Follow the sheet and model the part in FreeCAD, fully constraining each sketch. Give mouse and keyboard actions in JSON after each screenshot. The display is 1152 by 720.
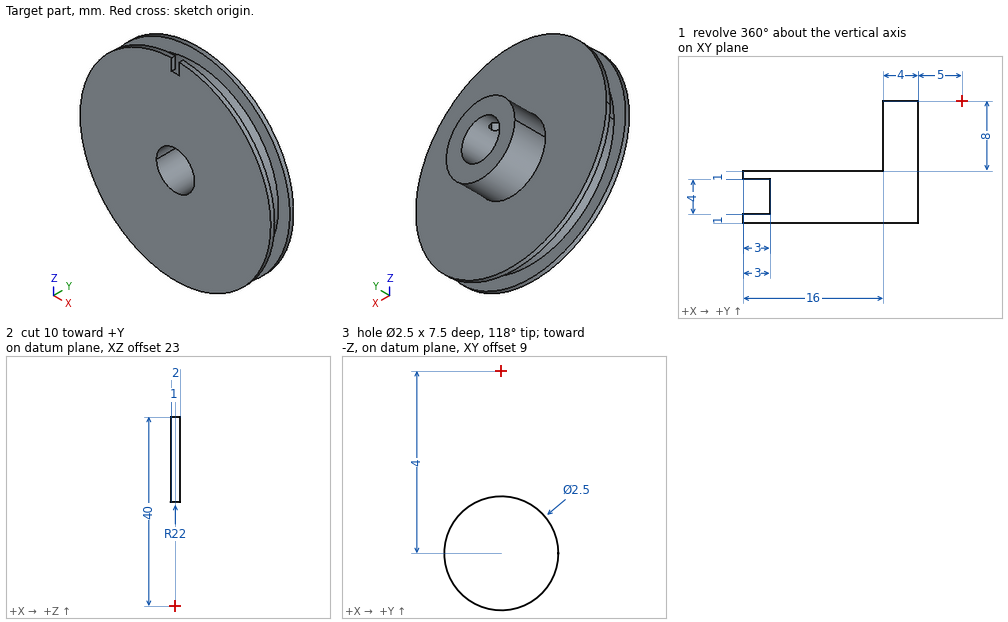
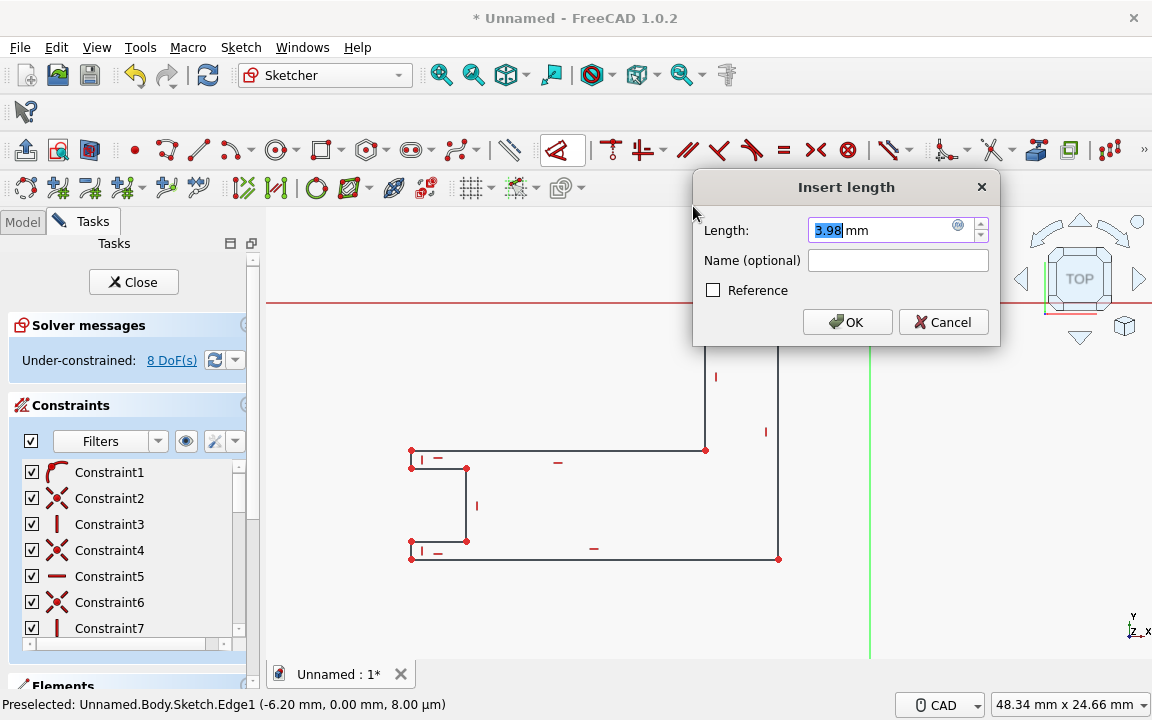
{"action": "type", "text": "4"}
{"action": "key", "text": "Return"}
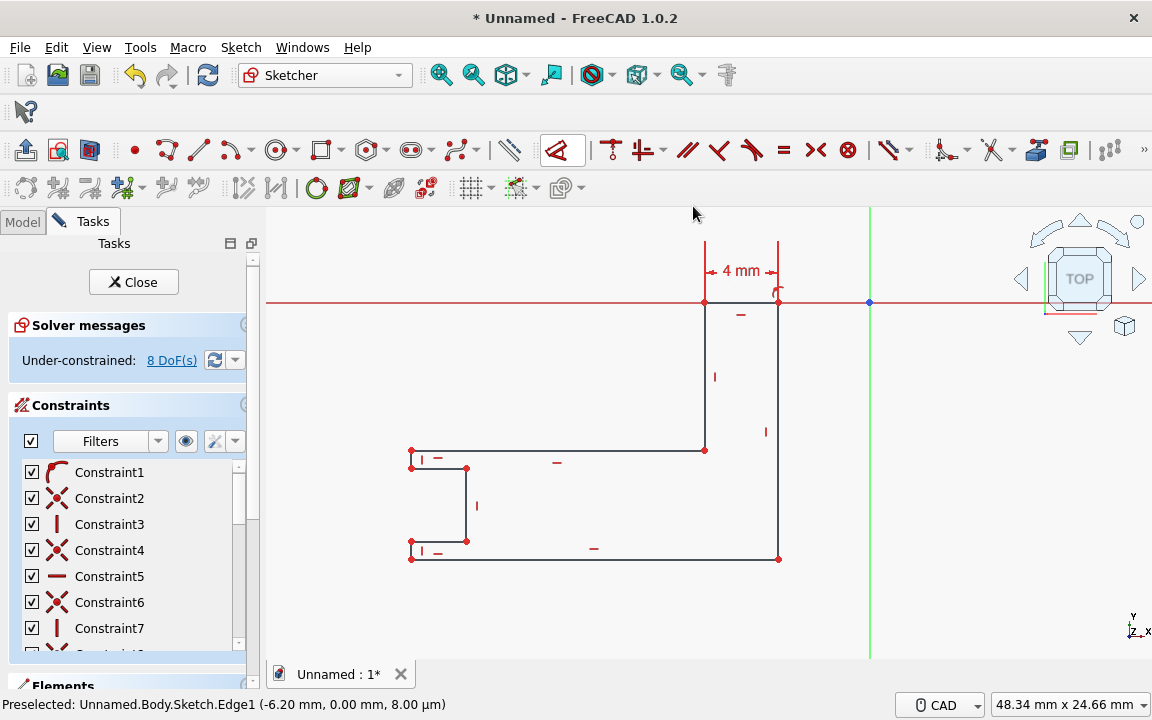
{"action": "left_click", "coordinate": [705, 347]}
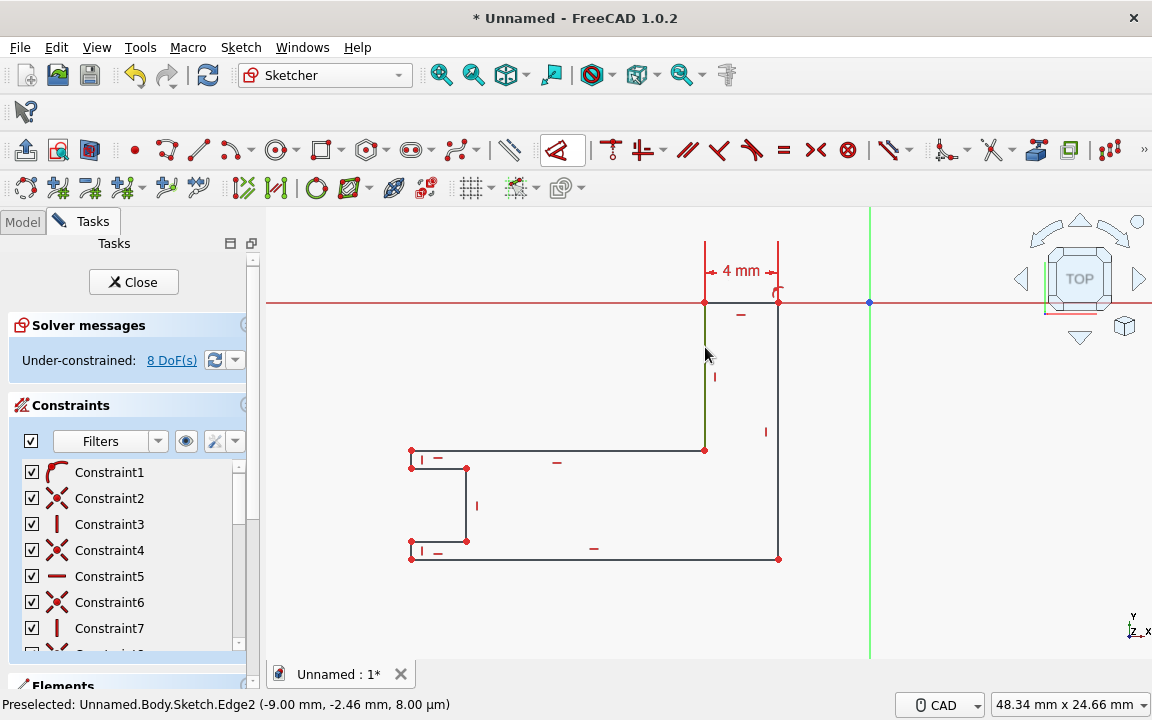
{"action": "key", "text": "i"}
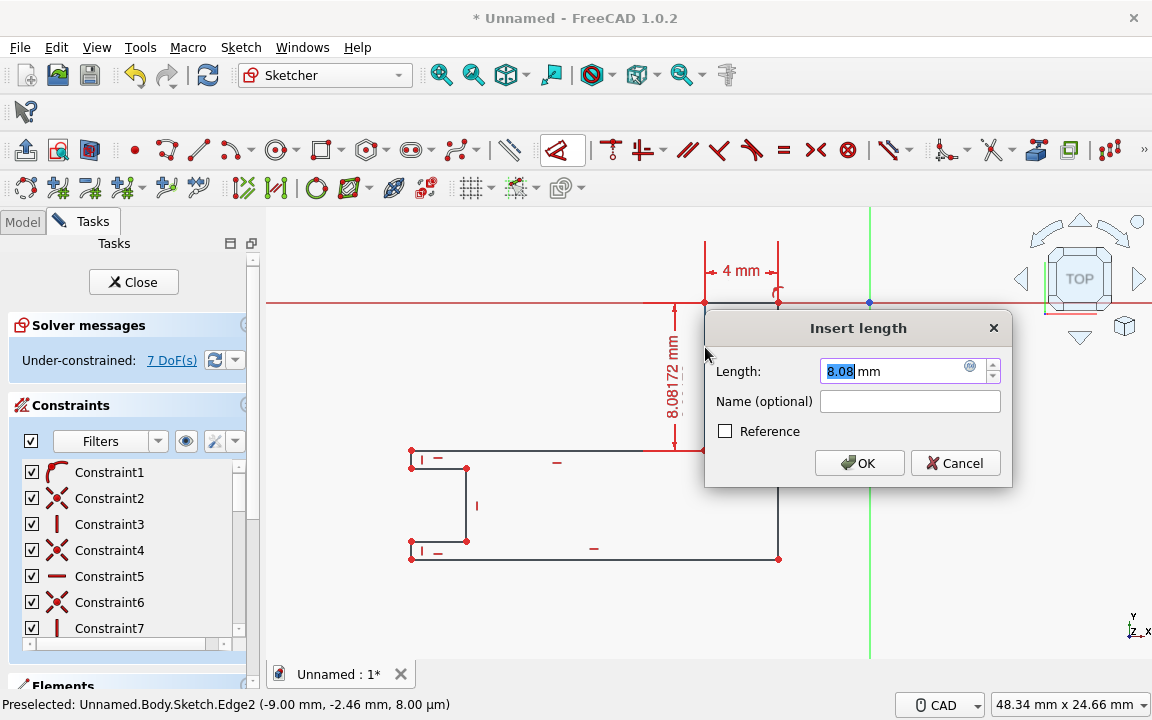
{"action": "type", "text": "8"}
{"action": "key", "text": "Return"}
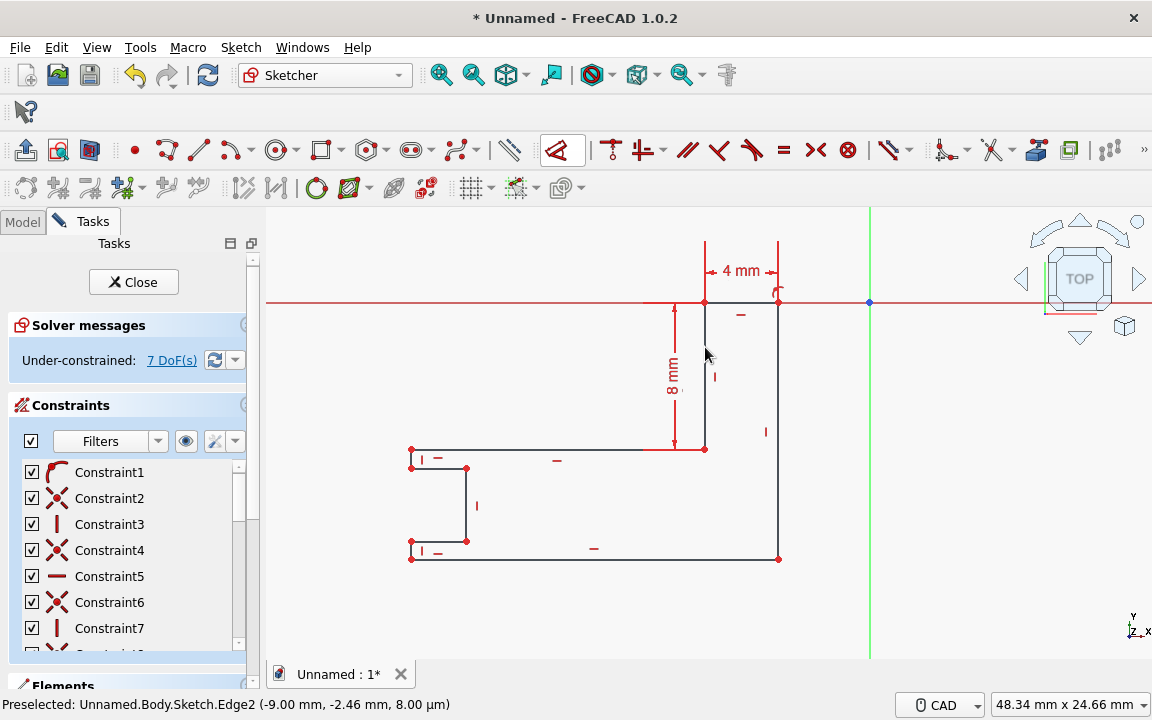
{"action": "scroll", "coordinate": [411, 459], "scroll_direction": "up", "scroll_amount": 4}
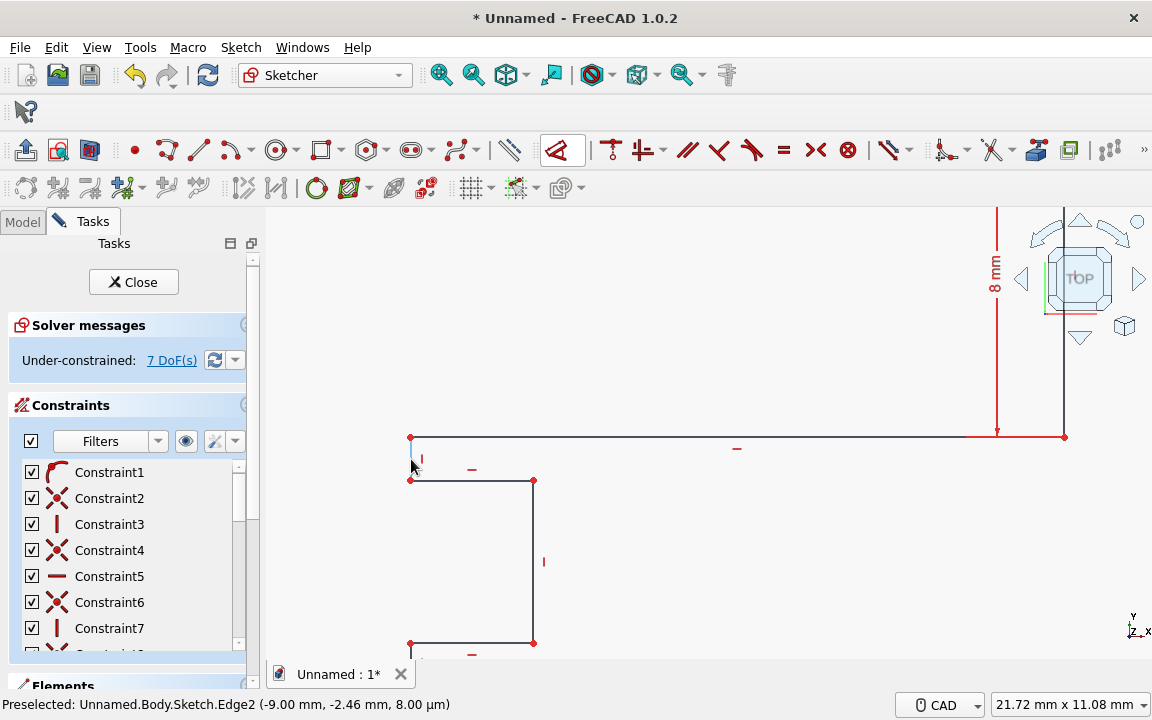
{"action": "left_click", "coordinate": [411, 459]}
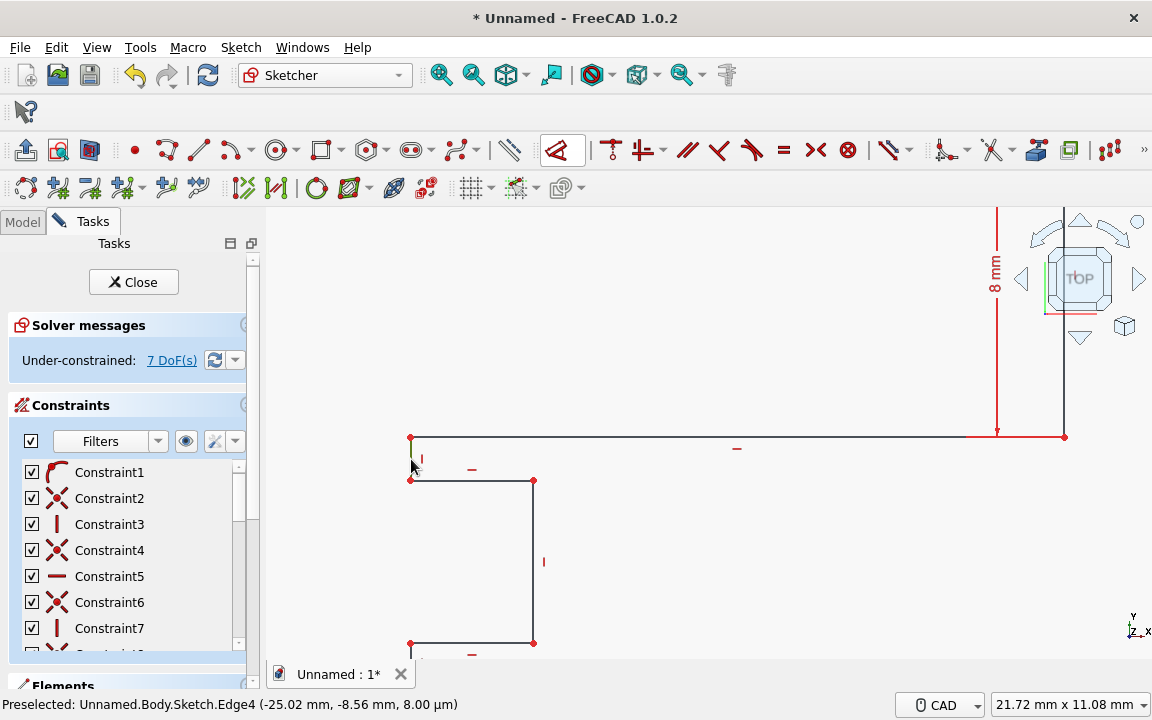
{"action": "key", "text": "i"}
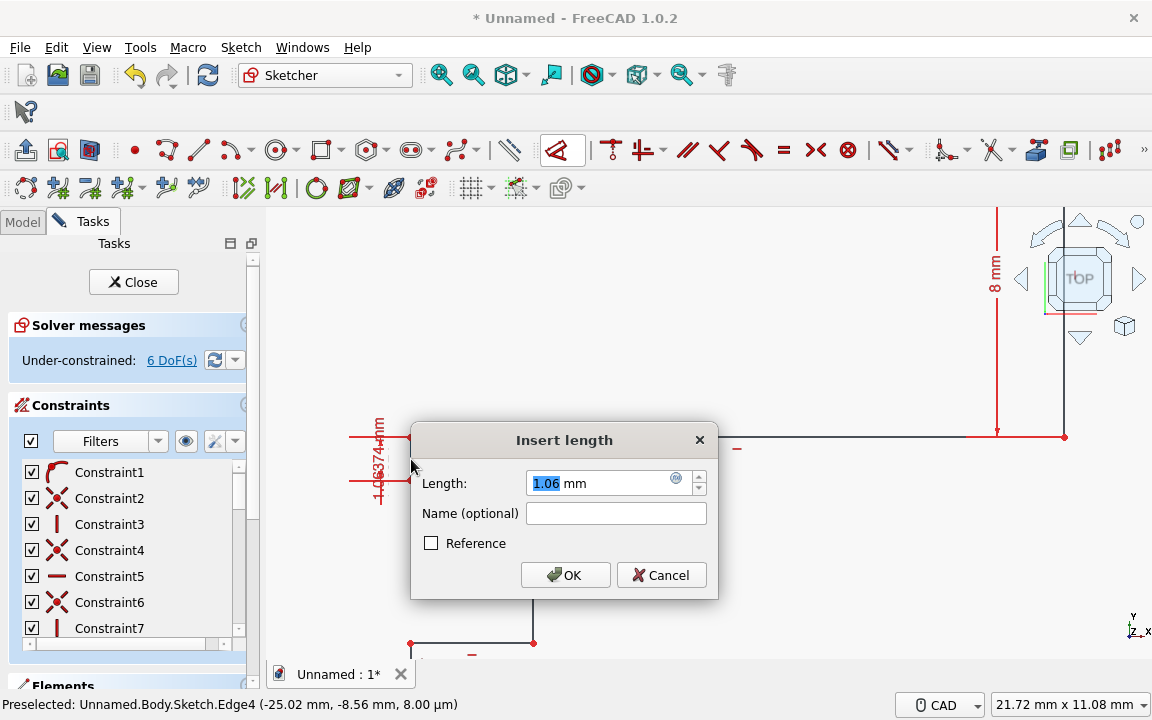
{"action": "type", "text": "1"}
{"action": "key", "text": "Return"}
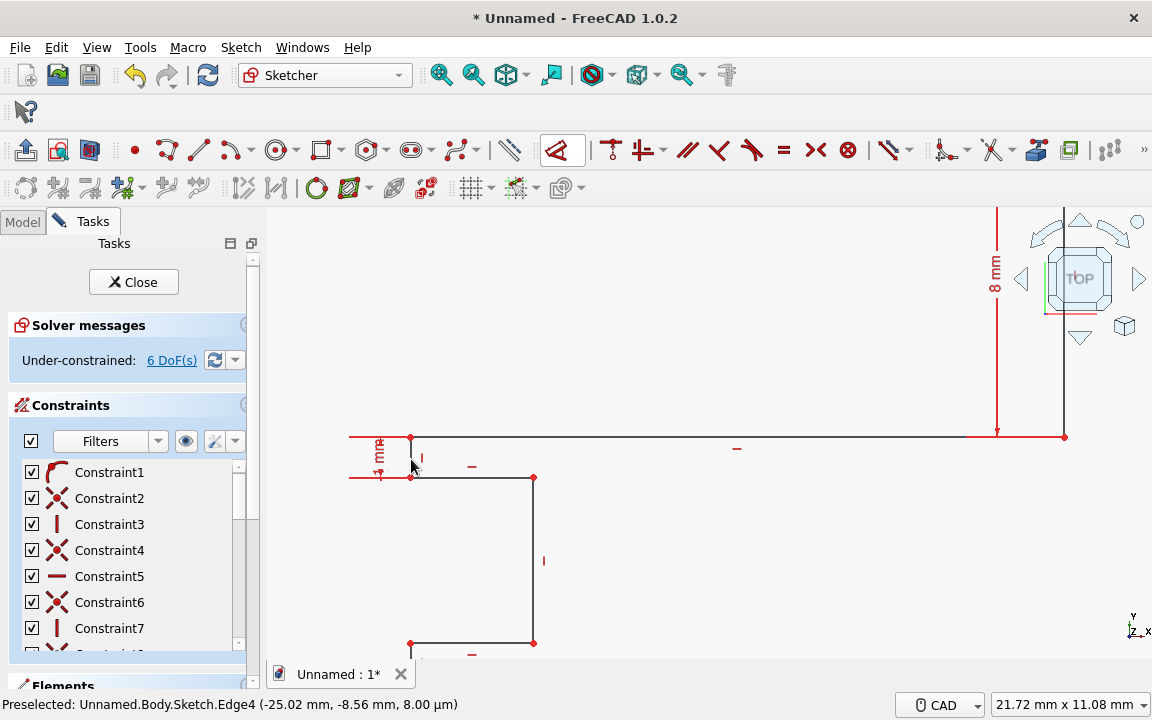
{"action": "left_click", "coordinate": [448, 478]}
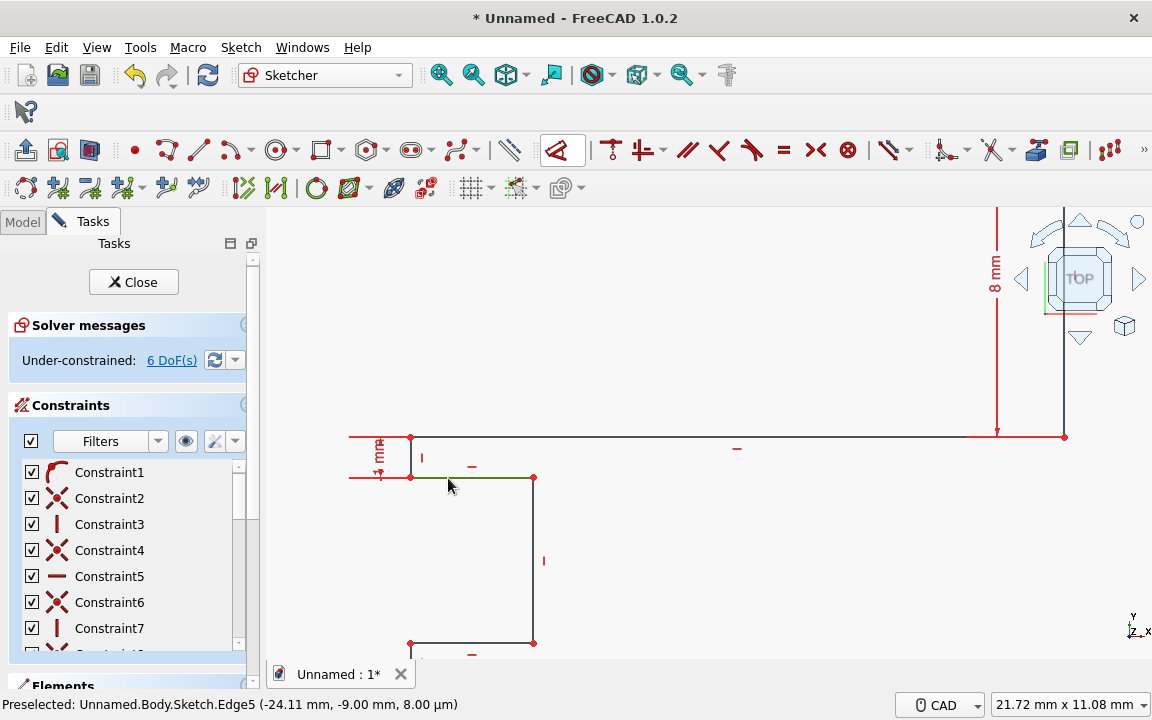
{"action": "key", "text": "l"}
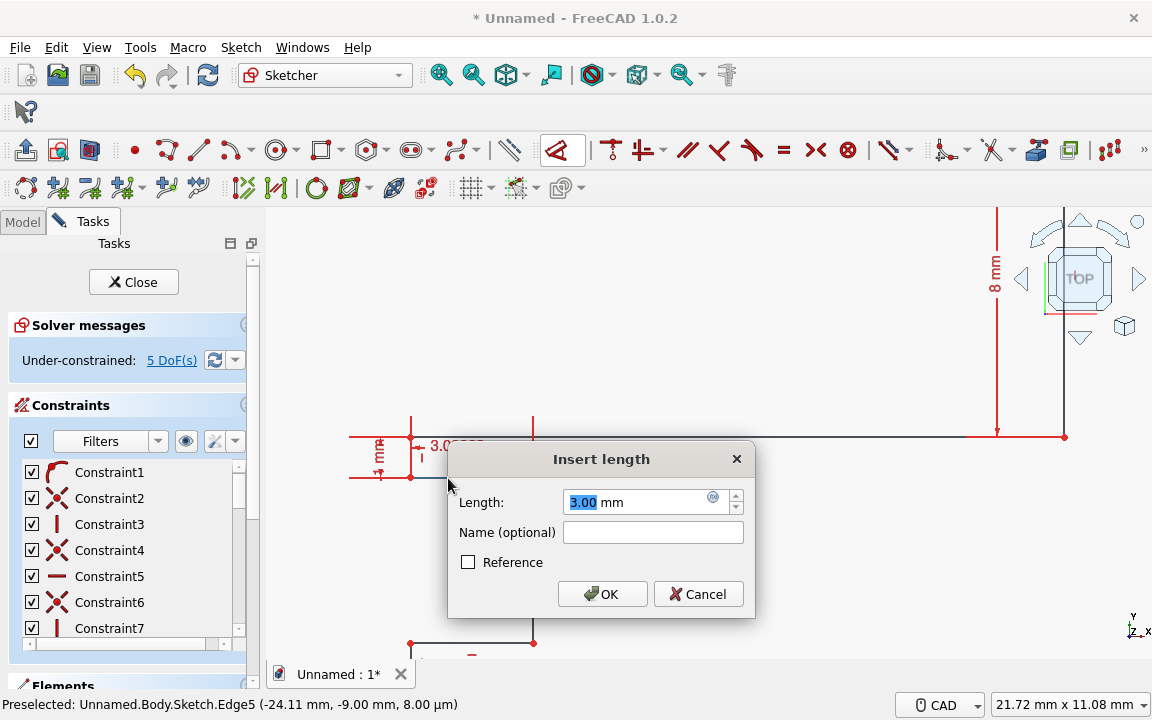
{"action": "type", "text": "3"}
{"action": "key", "text": "Return"}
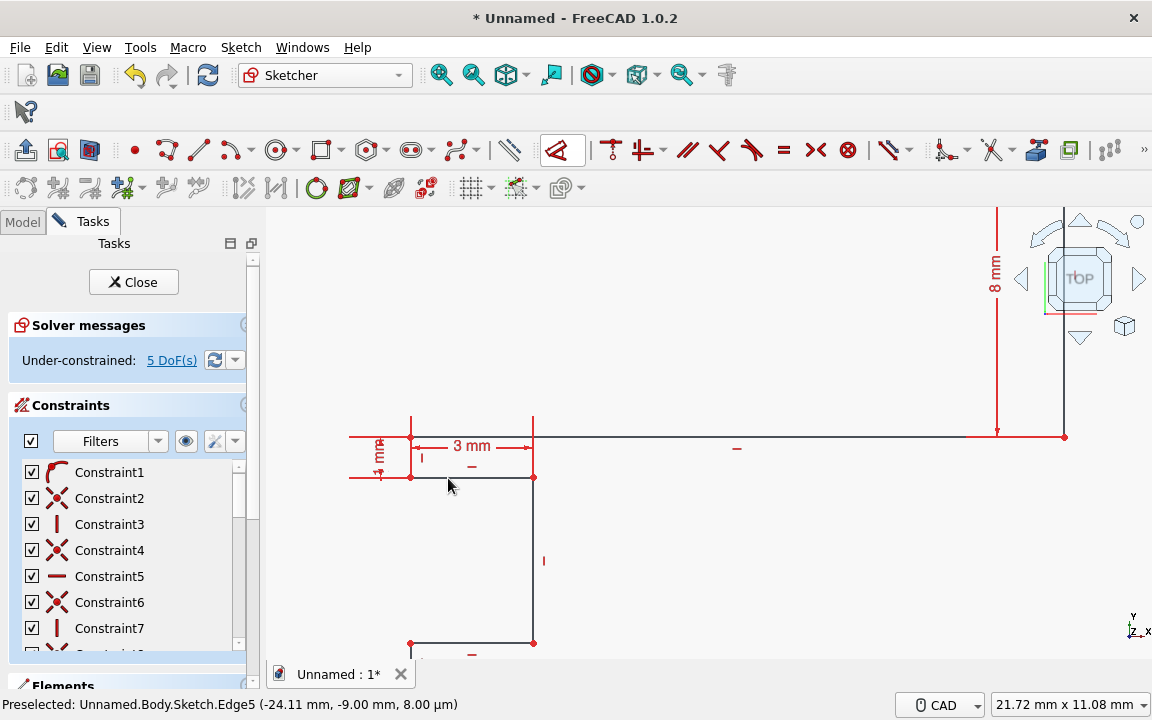
{"action": "left_click", "coordinate": [533, 527]}